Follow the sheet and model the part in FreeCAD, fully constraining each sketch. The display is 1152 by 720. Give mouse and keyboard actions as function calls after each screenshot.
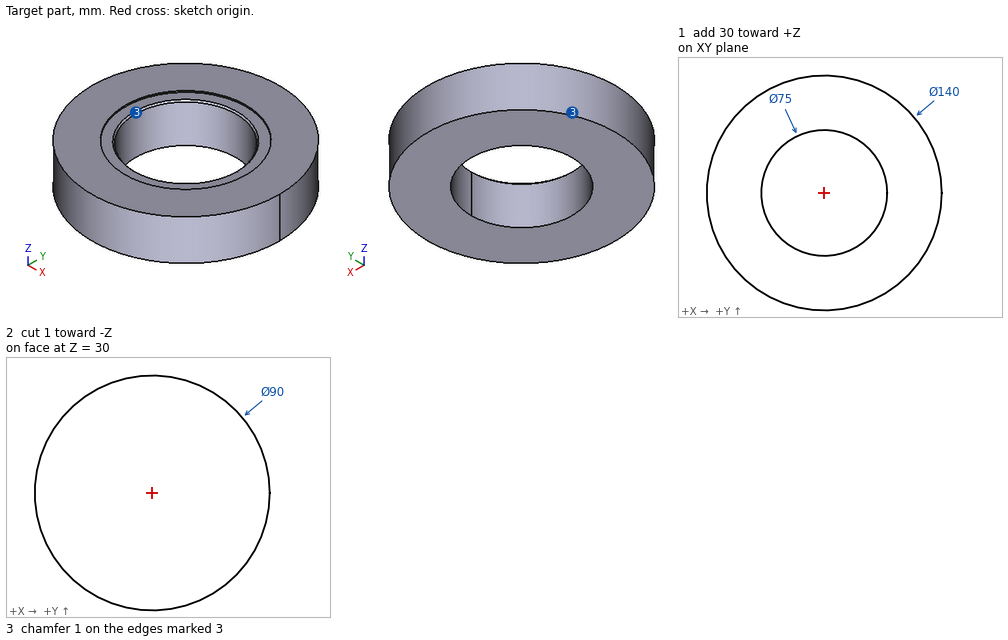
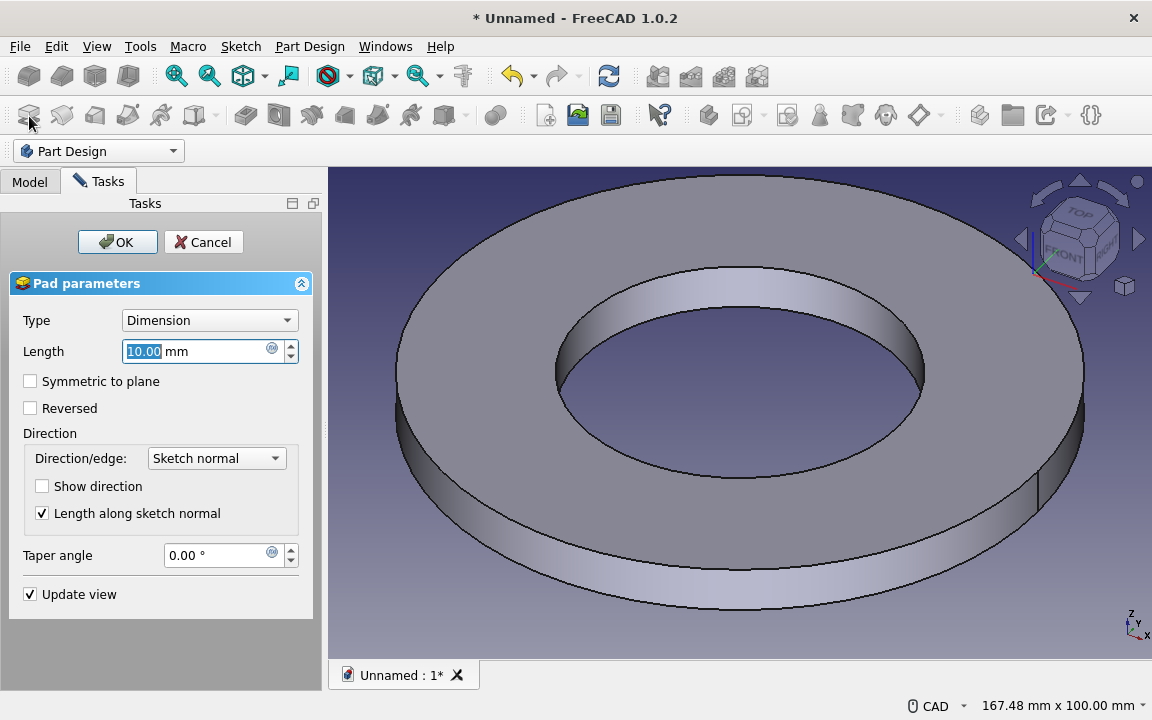
text(30)
key(Tab)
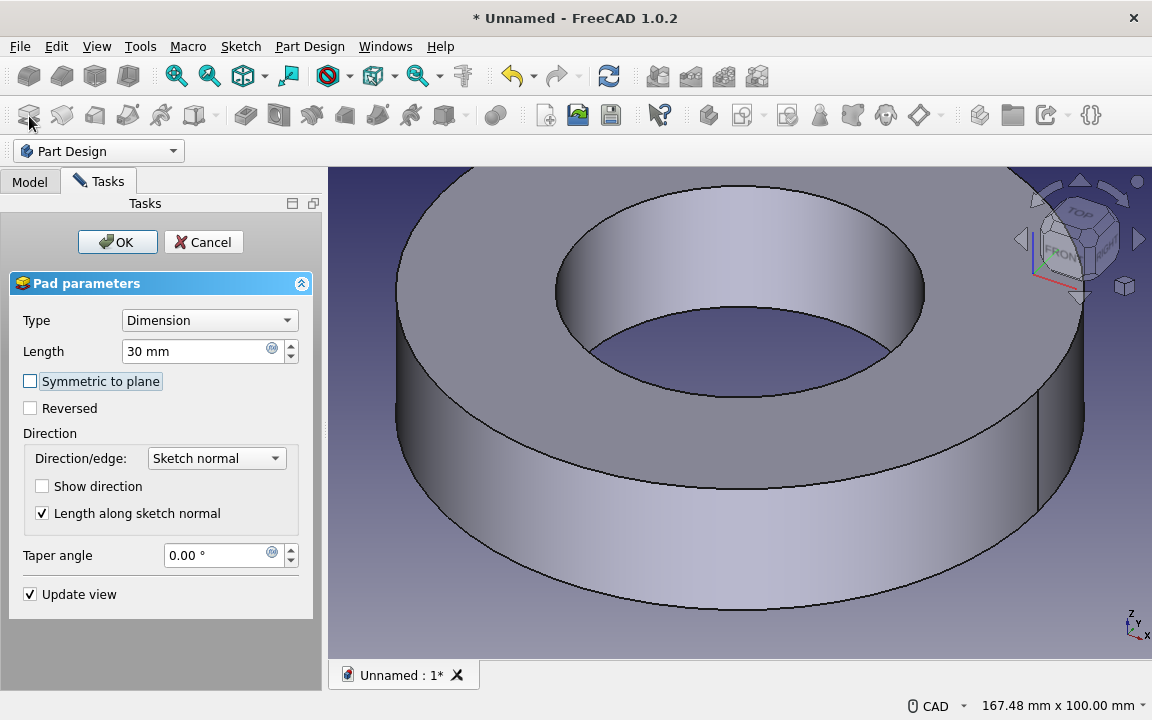
click(118, 242)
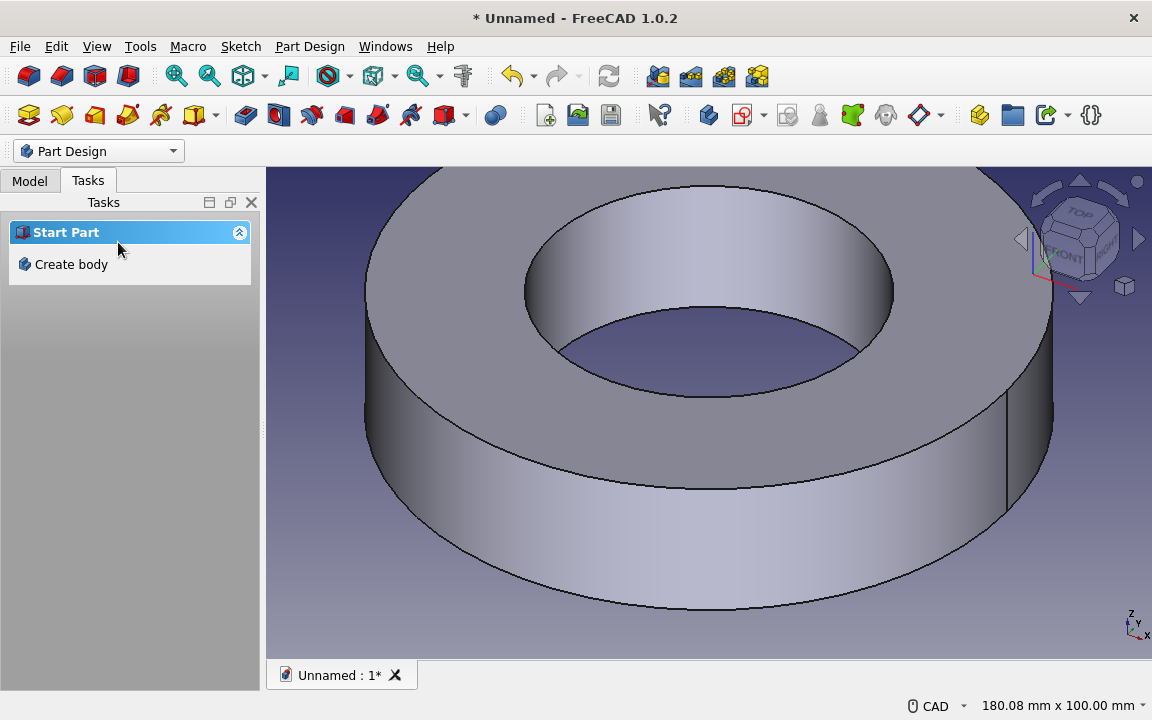
click(177, 76)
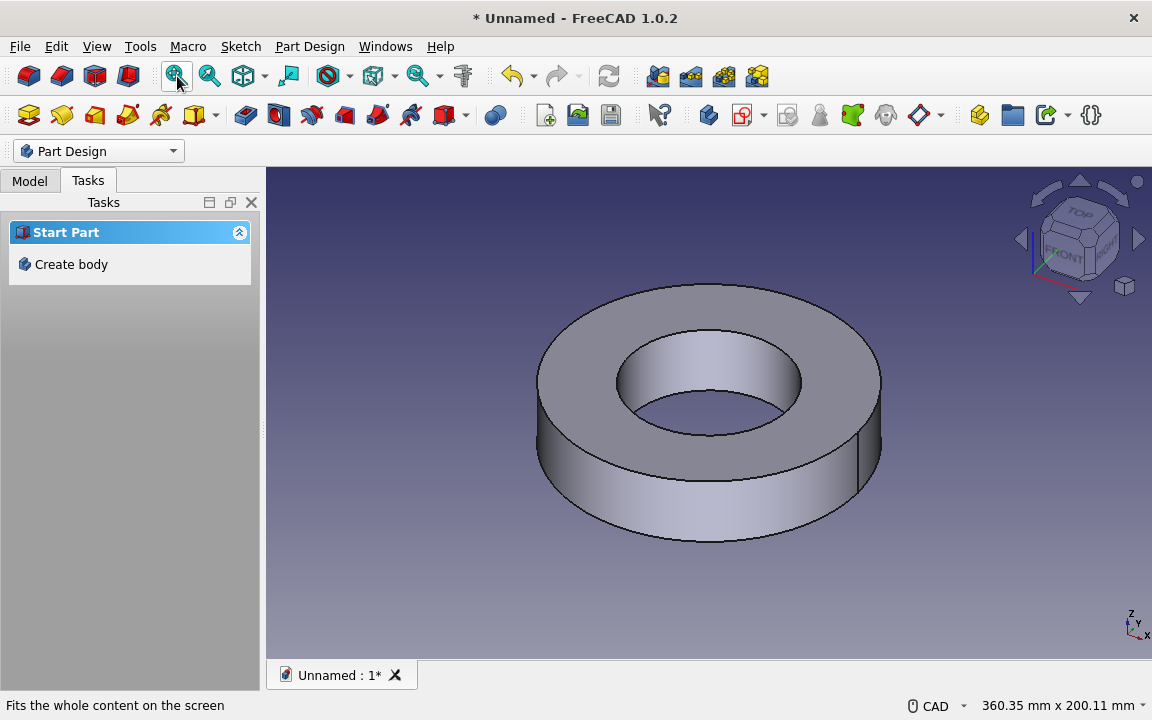
click(575, 402)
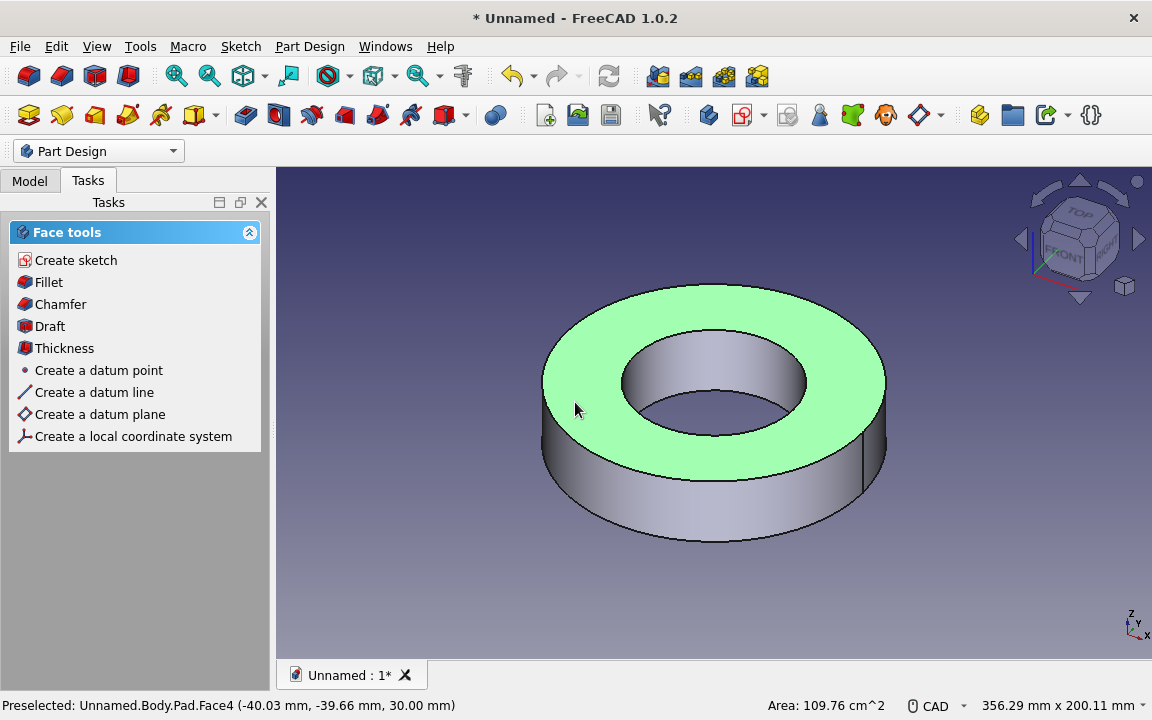
click(742, 116)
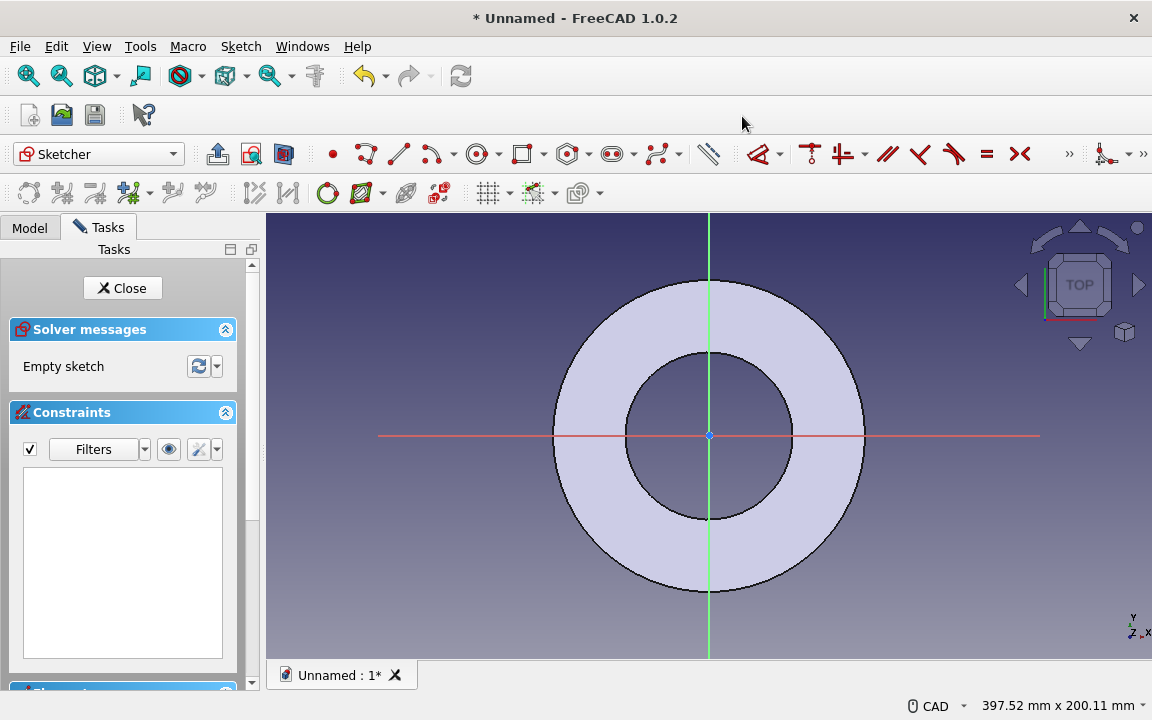
scroll(848, 436, up, 2)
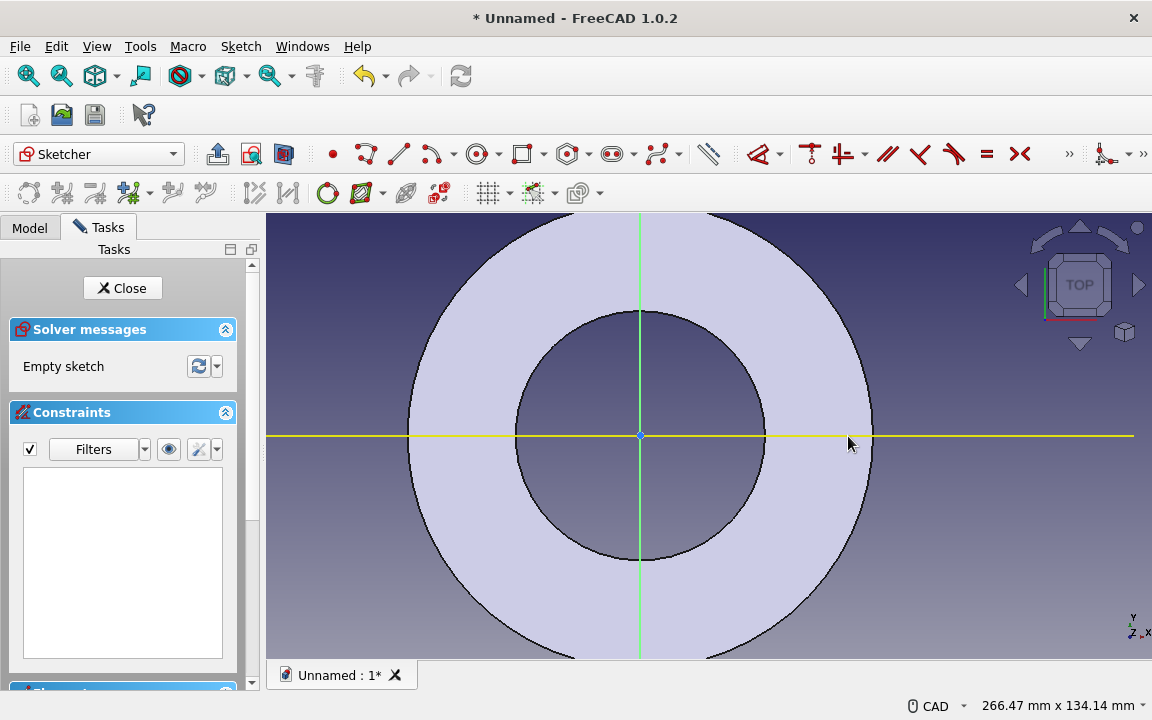
click(476, 154)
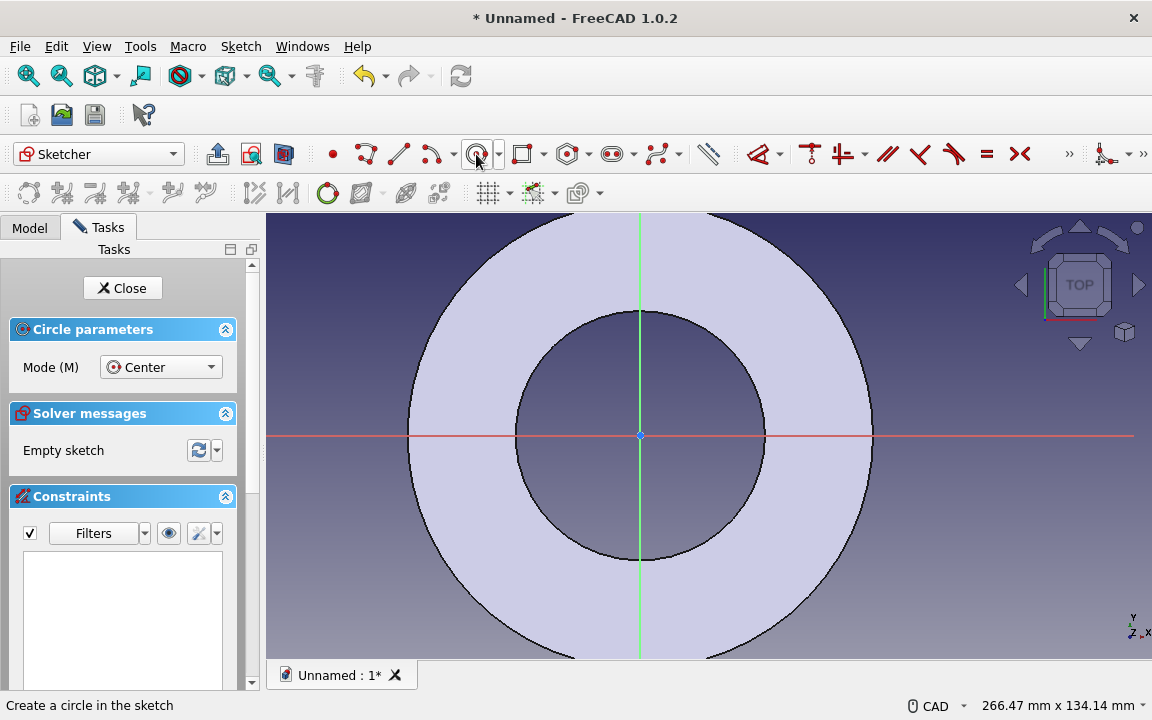
click(640, 436)
move(746, 330)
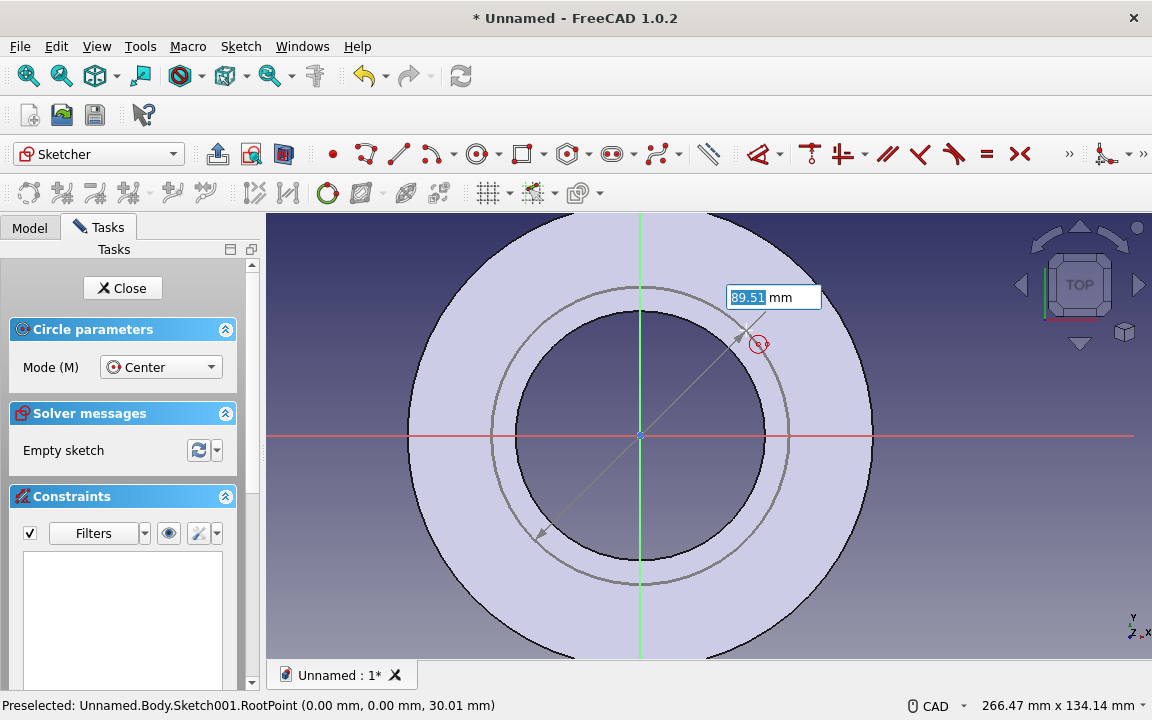
text(90)
key(Return)
key(Escape)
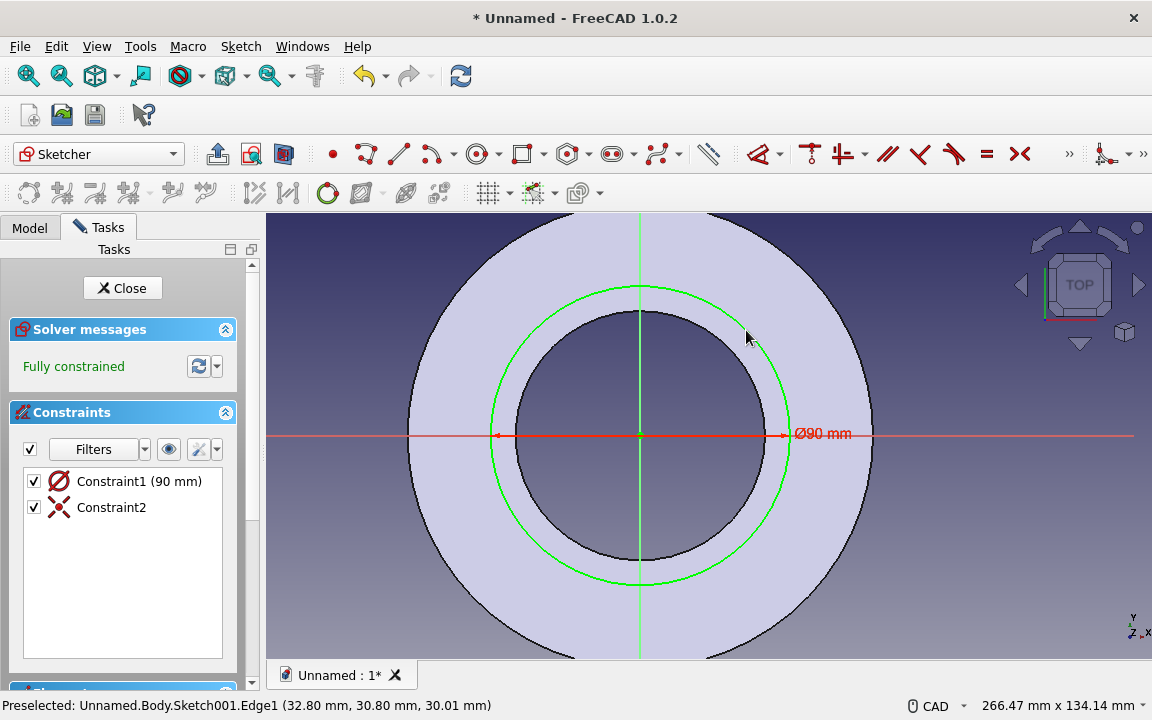
click(123, 288)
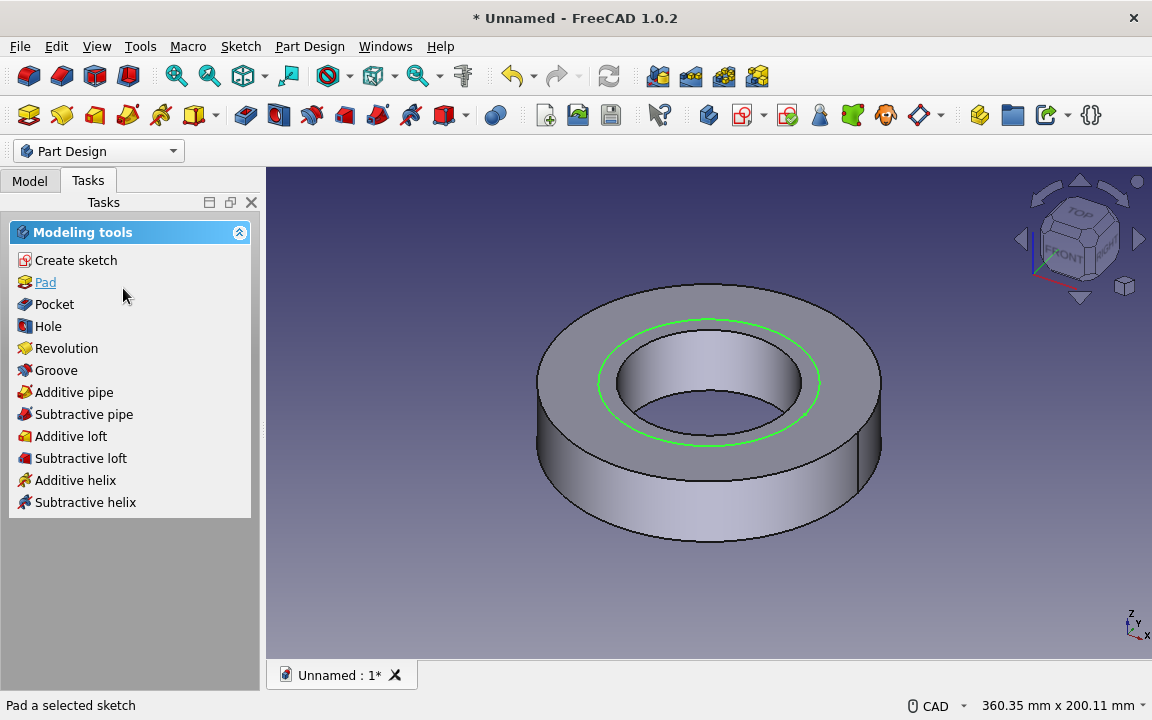
click(246, 116)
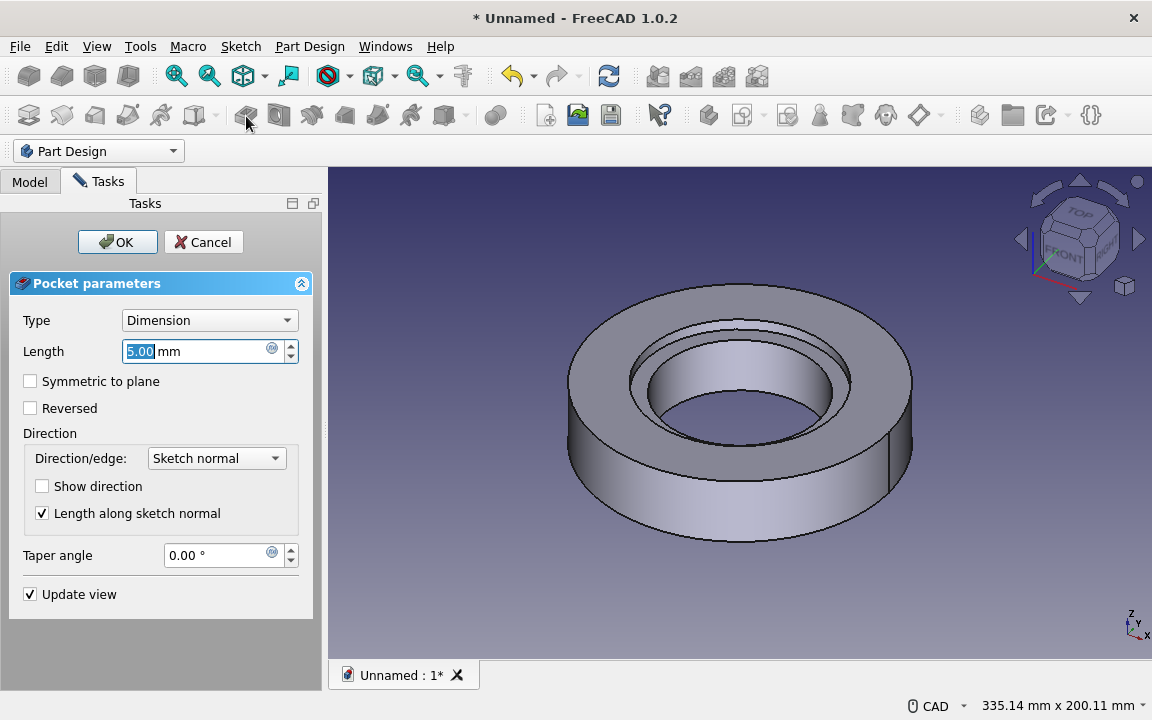
text(1)
key(Tab)